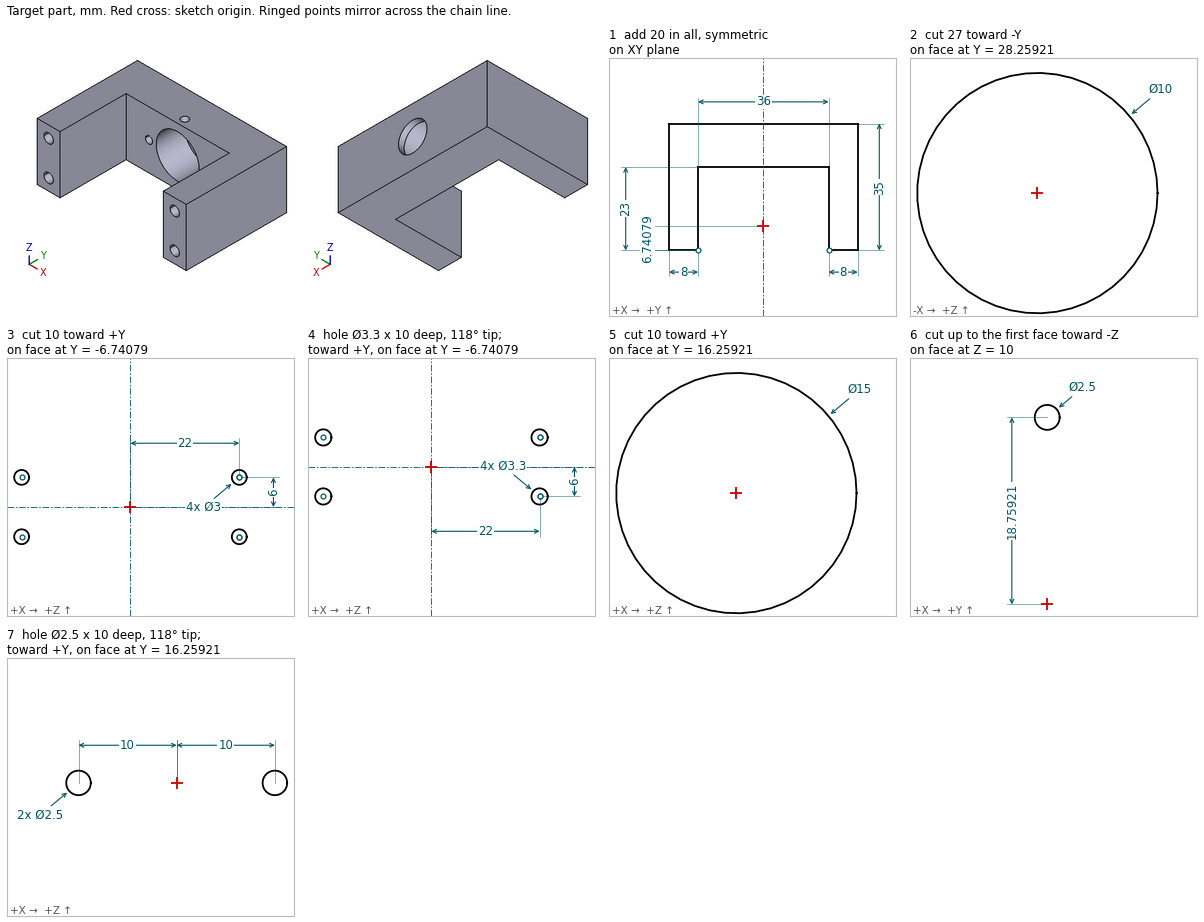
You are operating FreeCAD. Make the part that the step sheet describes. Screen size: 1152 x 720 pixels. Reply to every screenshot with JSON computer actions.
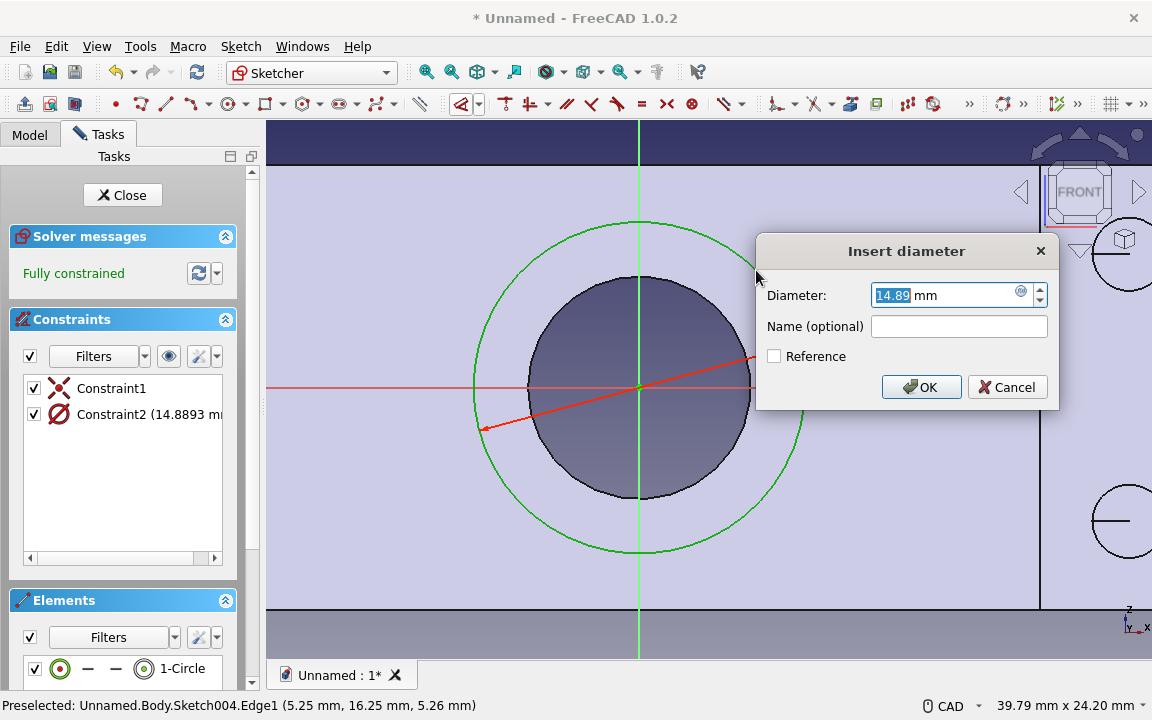
{"action": "type", "text": "15"}
{"action": "key", "text": "Return"}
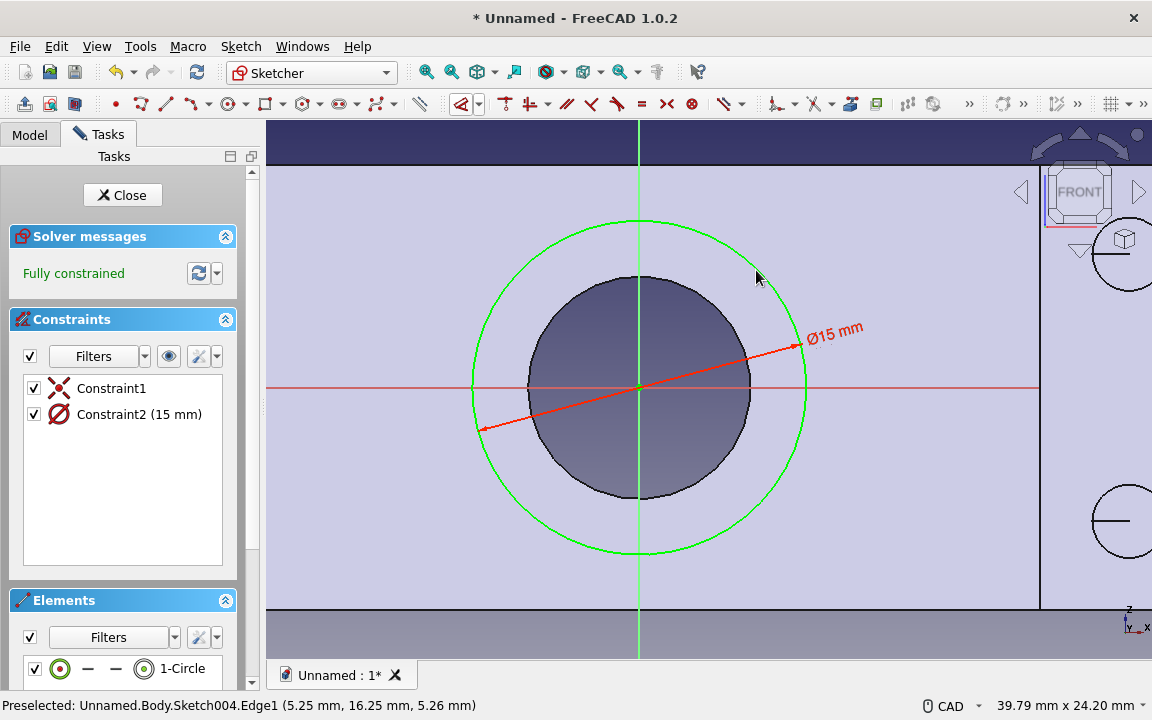
{"action": "left_click", "coordinate": [123, 195]}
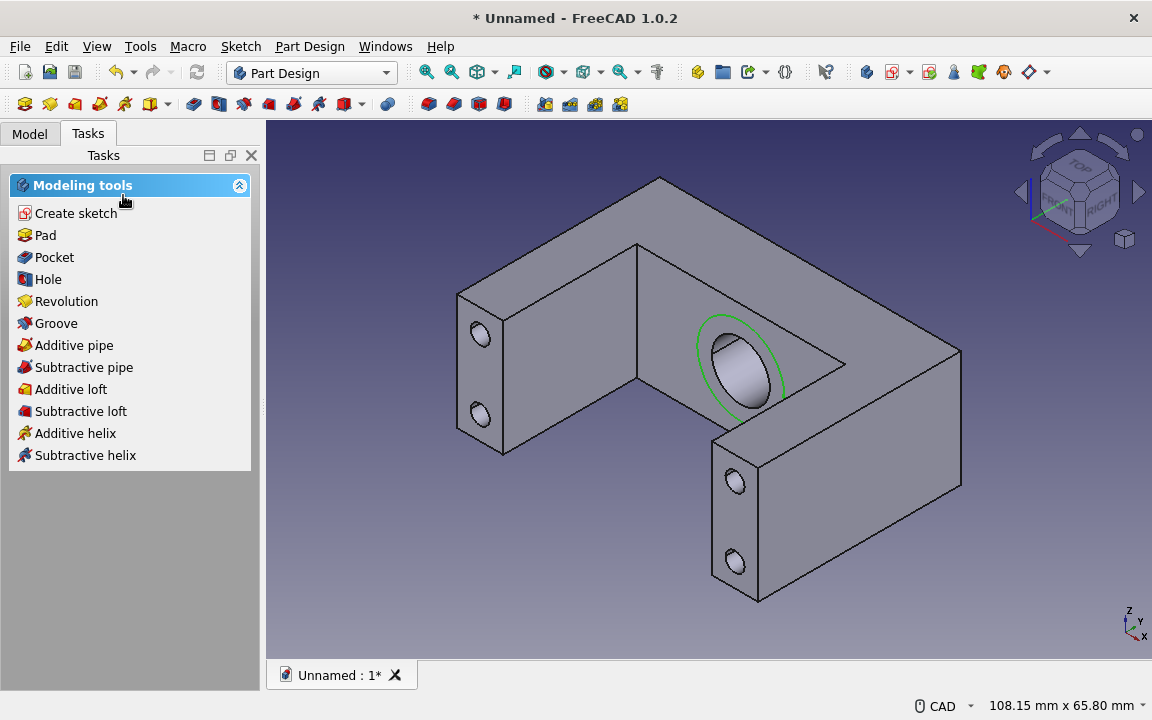
{"action": "left_click", "coordinate": [194, 104]}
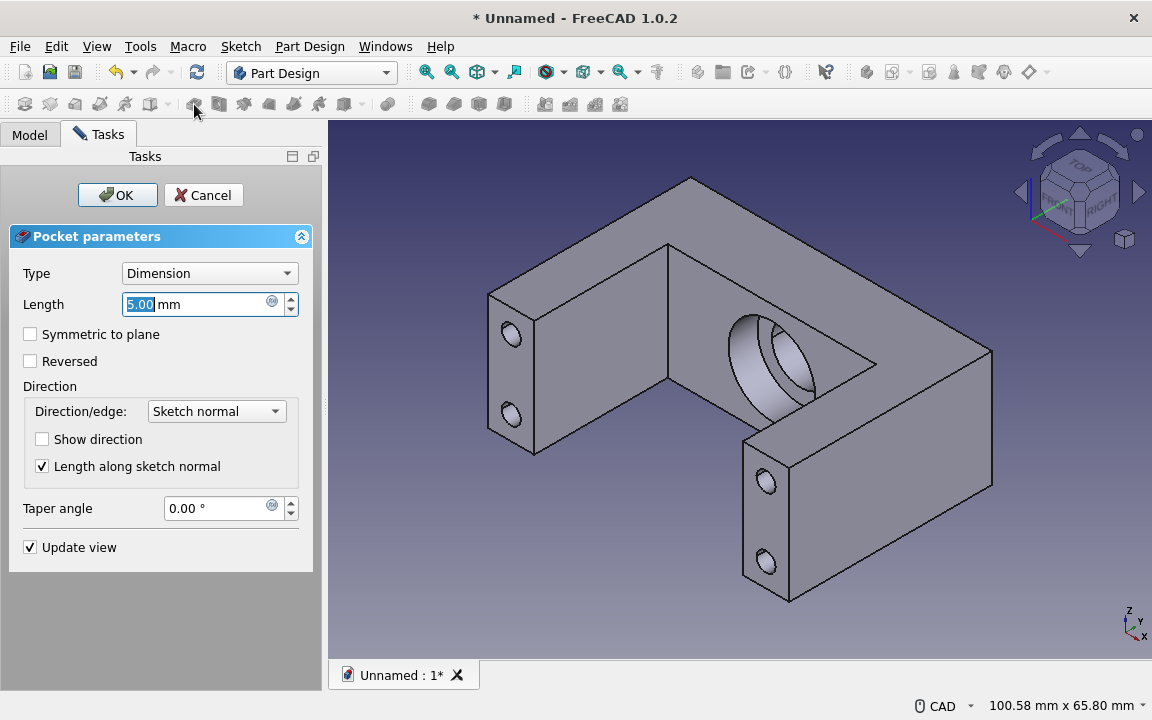
{"action": "type", "text": "10"}
{"action": "key", "text": "Tab"}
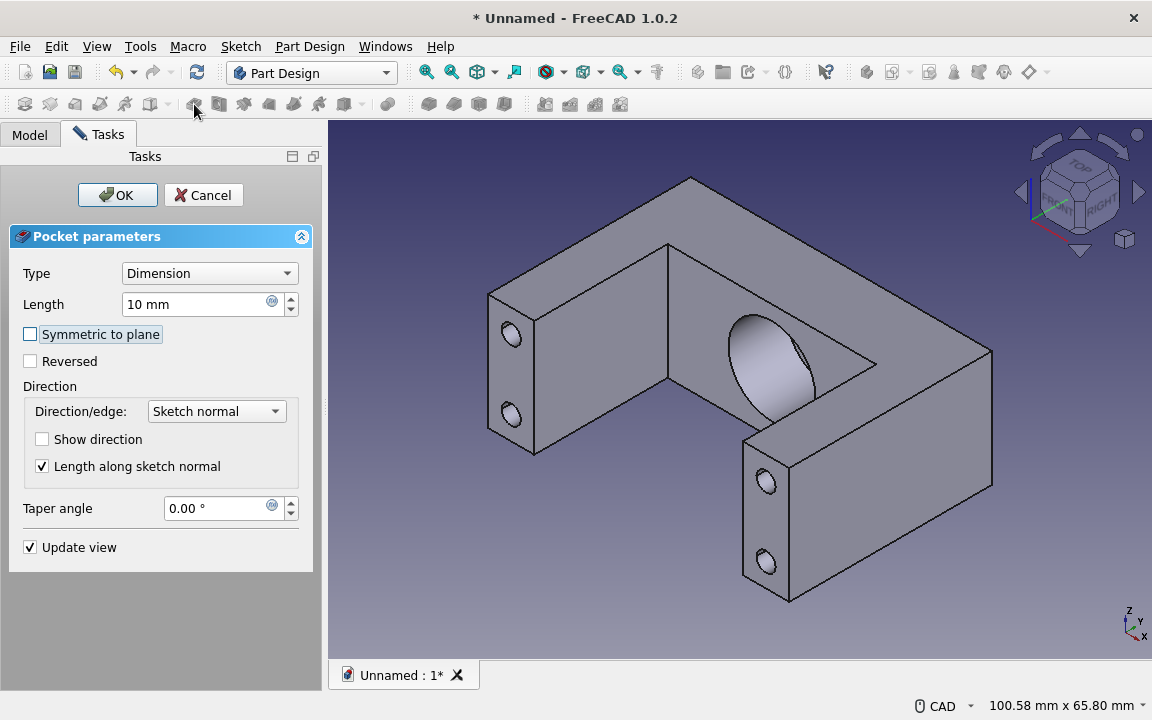
{"action": "left_click", "coordinate": [118, 195]}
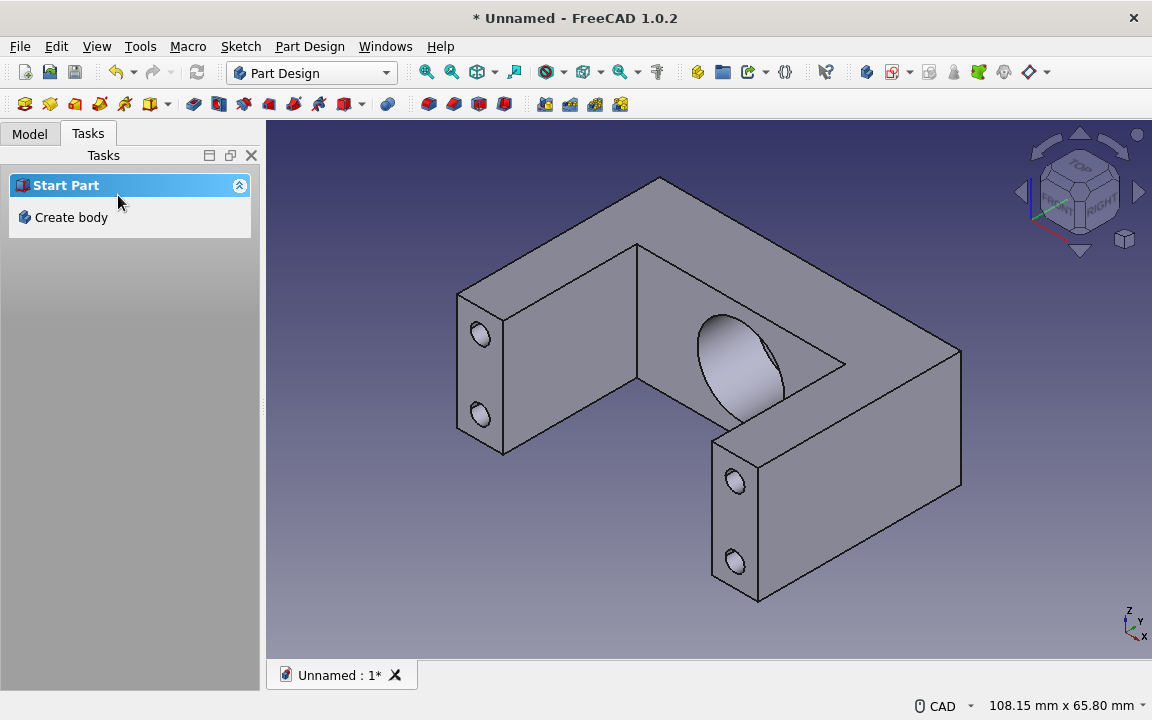
{"action": "left_click", "coordinate": [853, 338]}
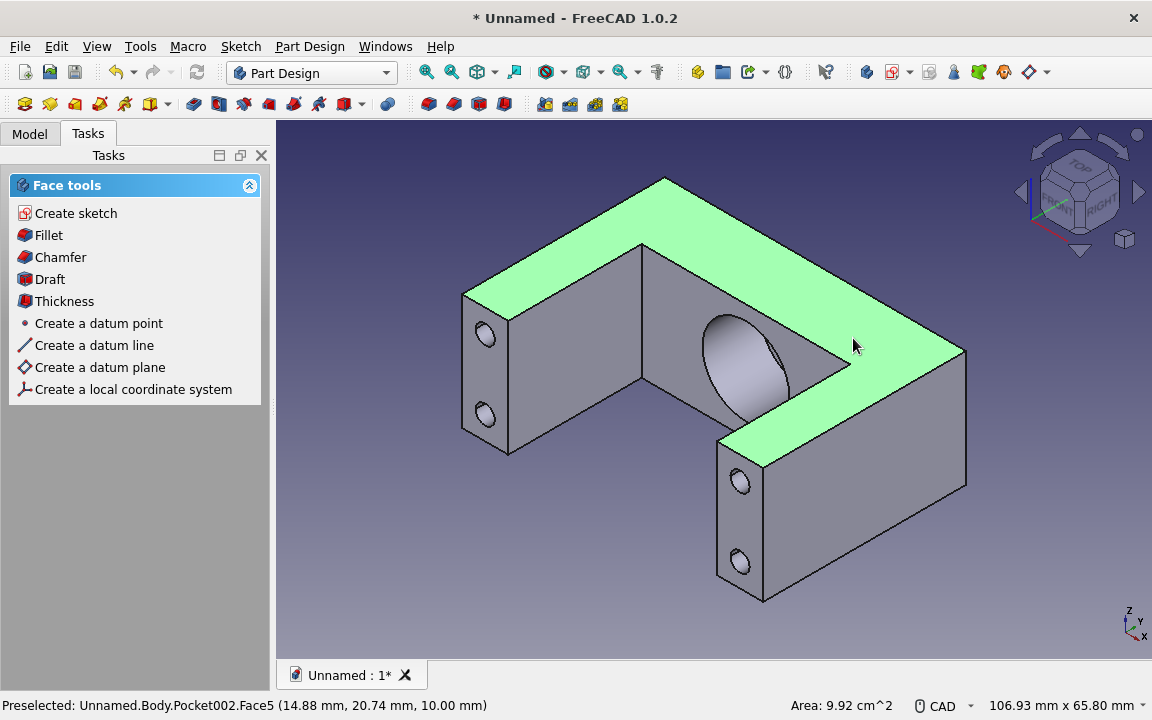
{"action": "left_click", "coordinate": [892, 72]}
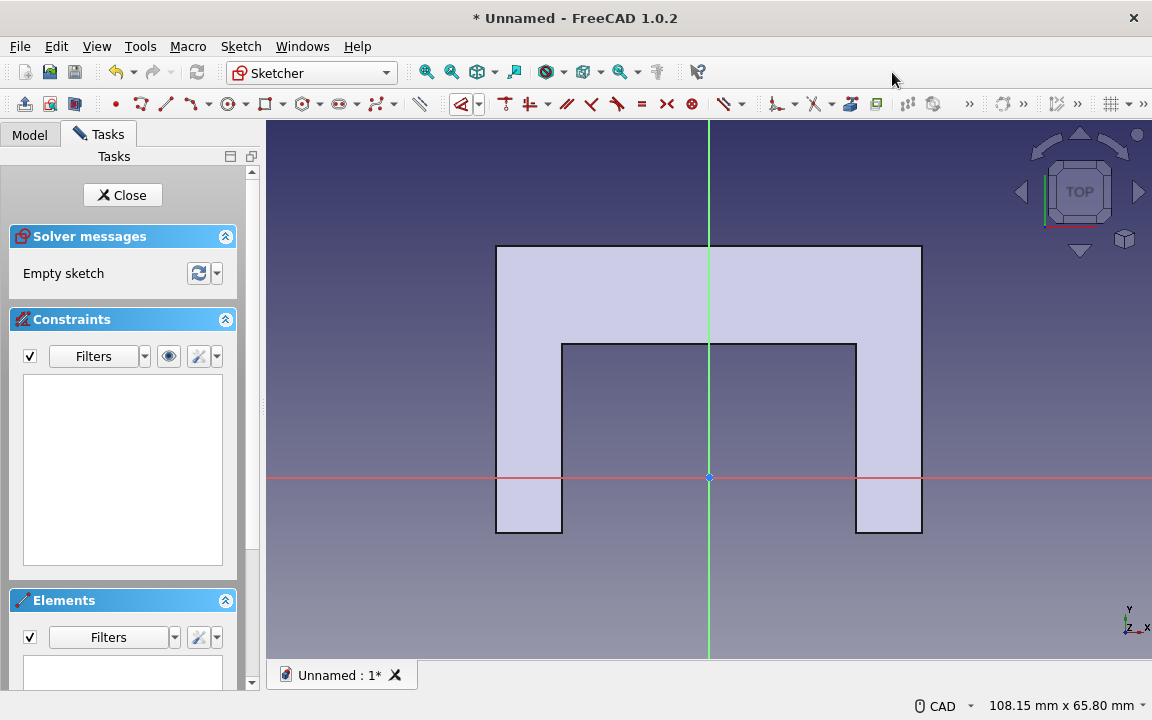
{"action": "scroll", "coordinate": [713, 320], "scroll_direction": "up", "scroll_amount": 14}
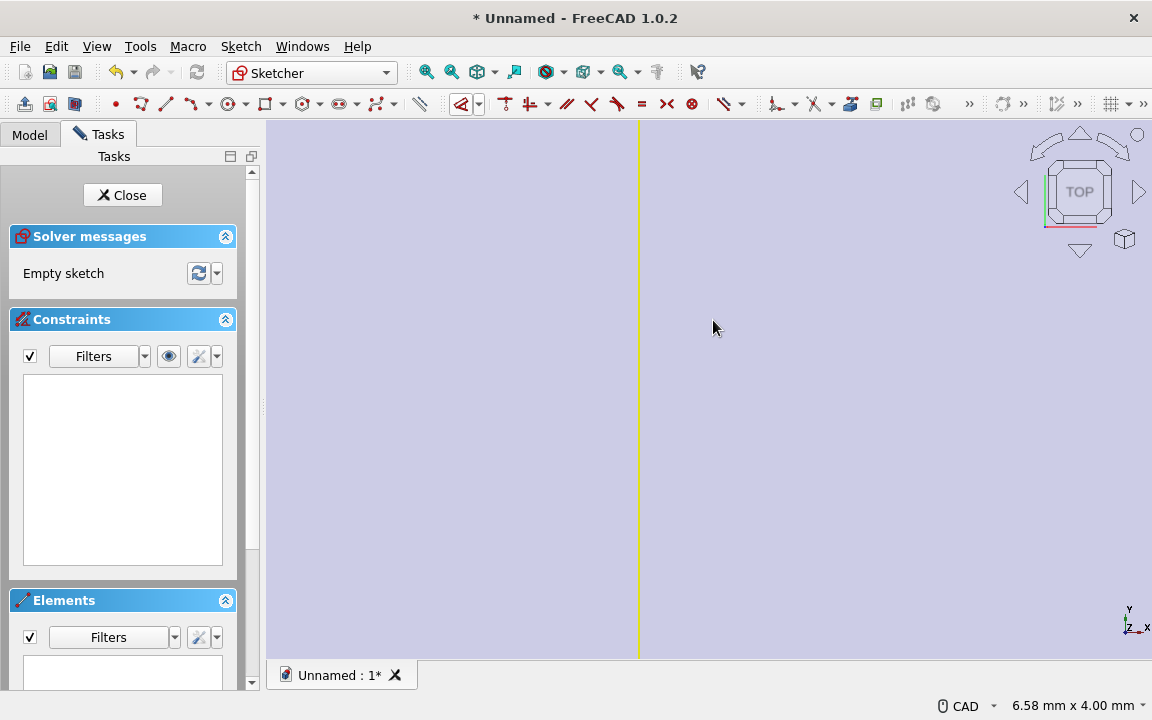
{"action": "left_click", "coordinate": [228, 104]}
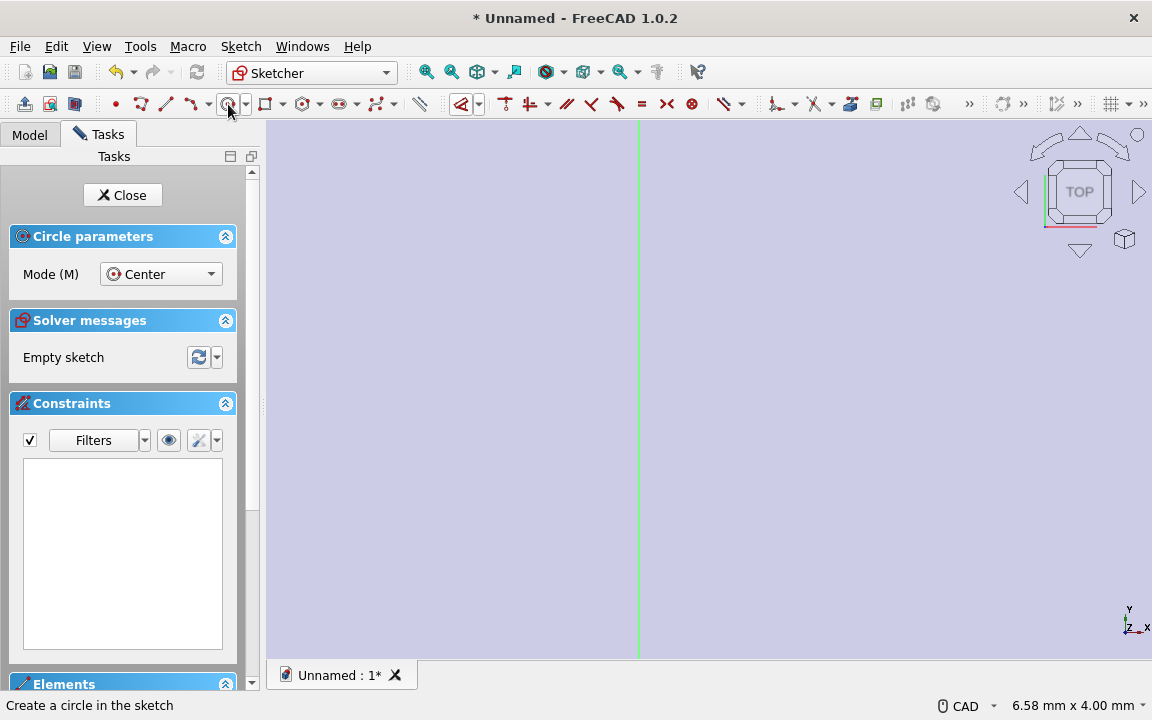
{"action": "left_click", "coordinate": [639, 379]}
{"action": "left_click", "coordinate": [758, 260]}
{"action": "key", "text": "Escape"}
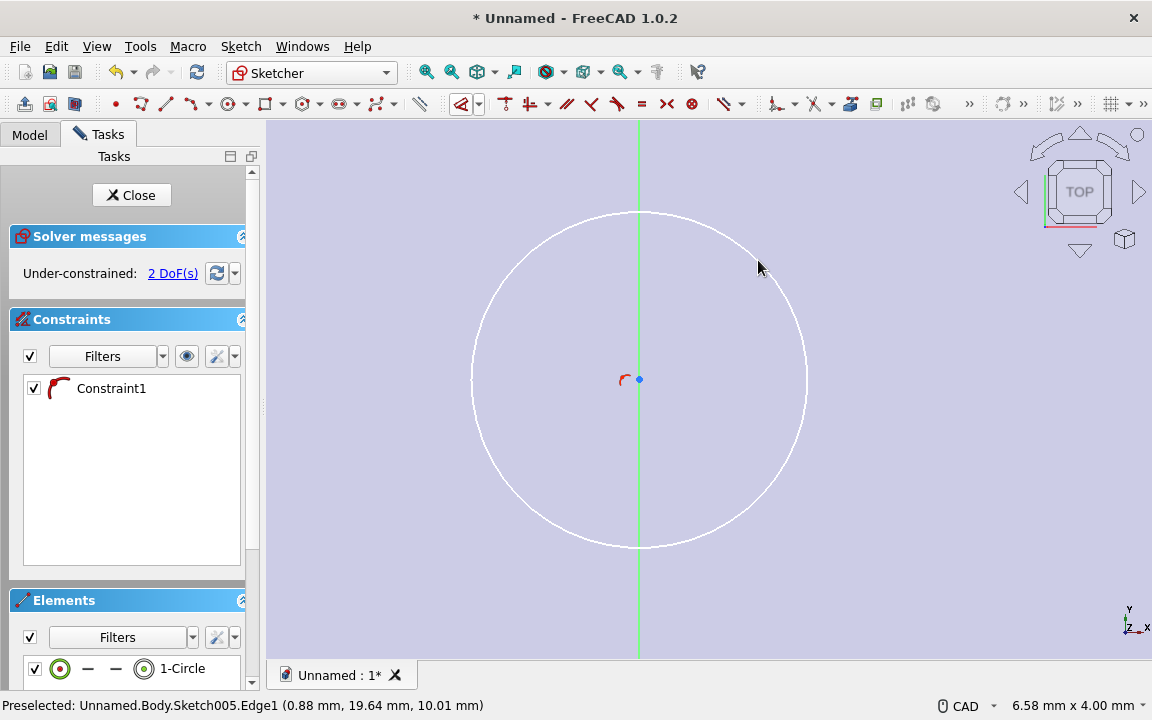
{"action": "left_click", "coordinate": [758, 261]}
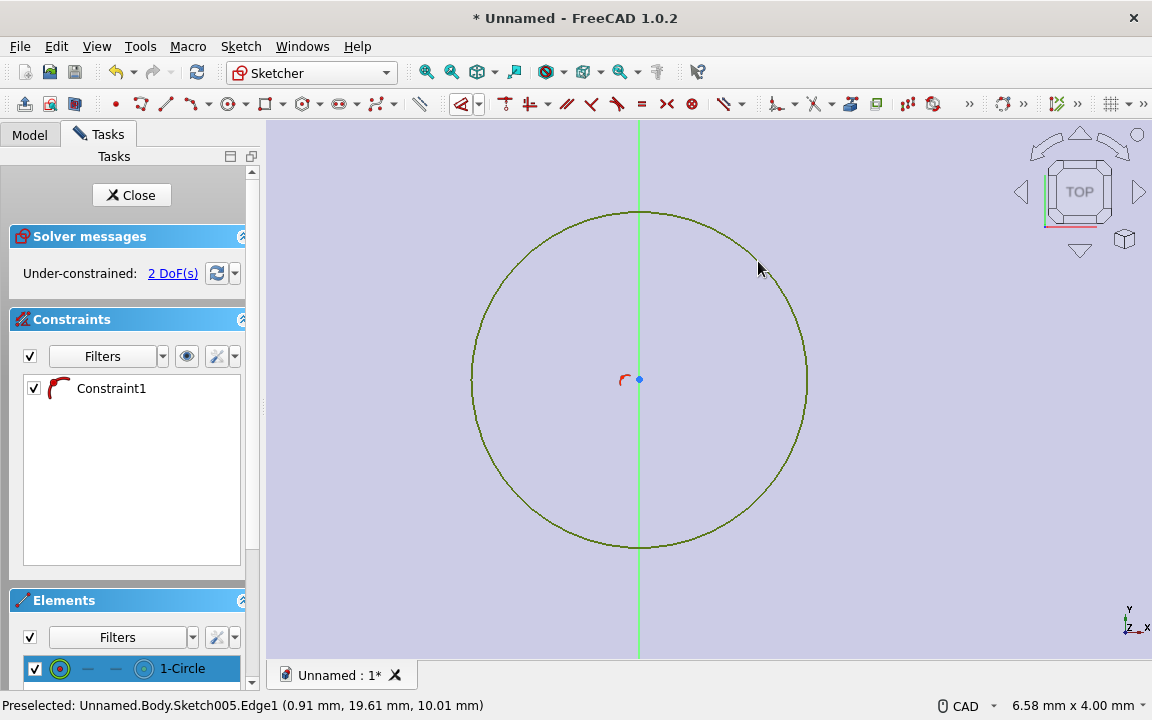
{"action": "key", "text": "k o"}